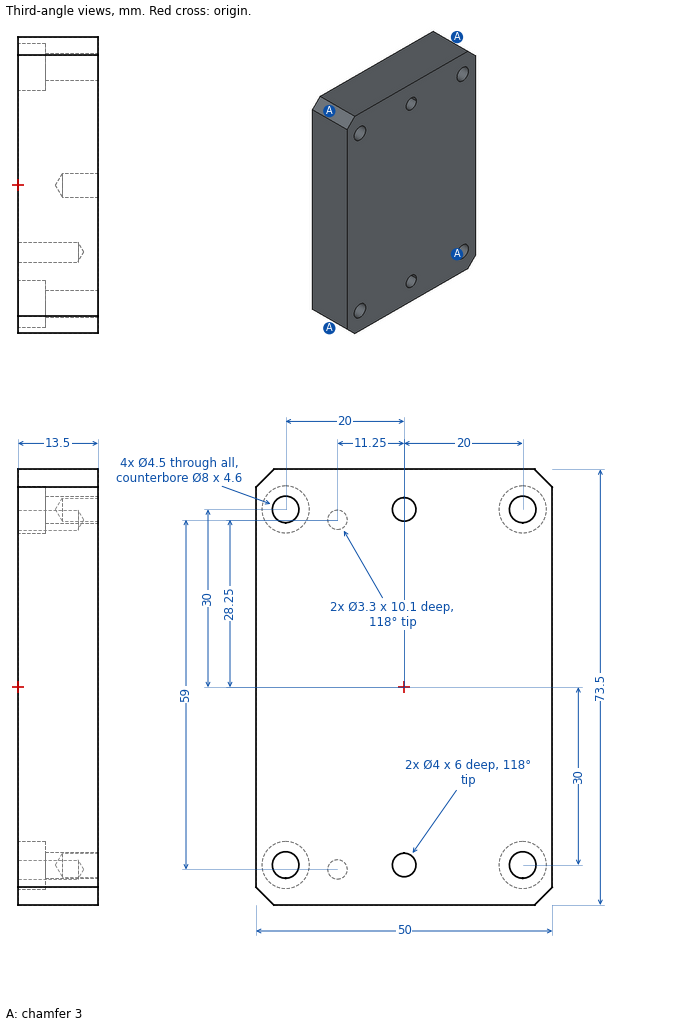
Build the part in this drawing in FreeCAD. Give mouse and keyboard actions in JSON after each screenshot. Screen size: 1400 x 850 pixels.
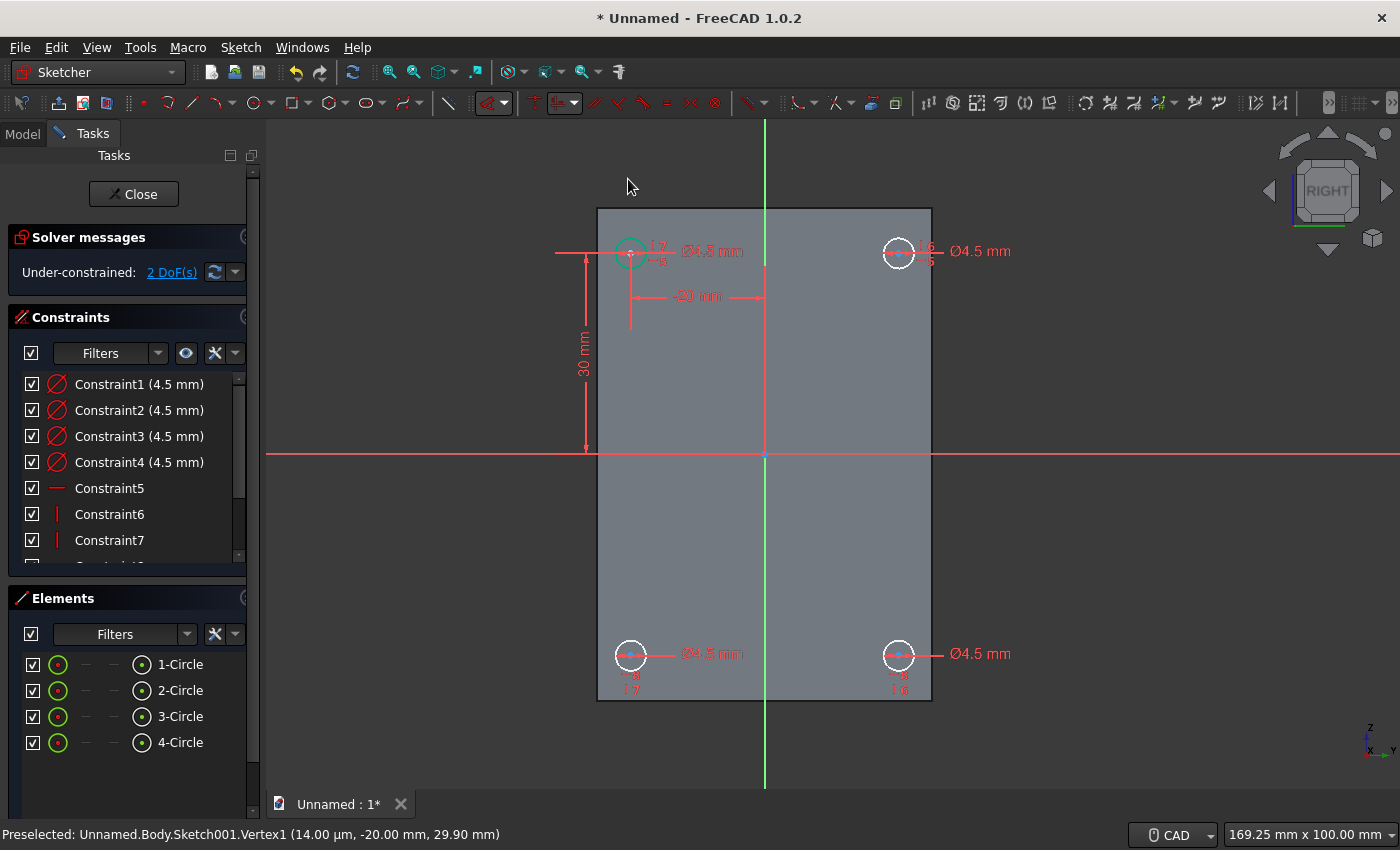
{"action": "left_click", "coordinate": [899, 253]}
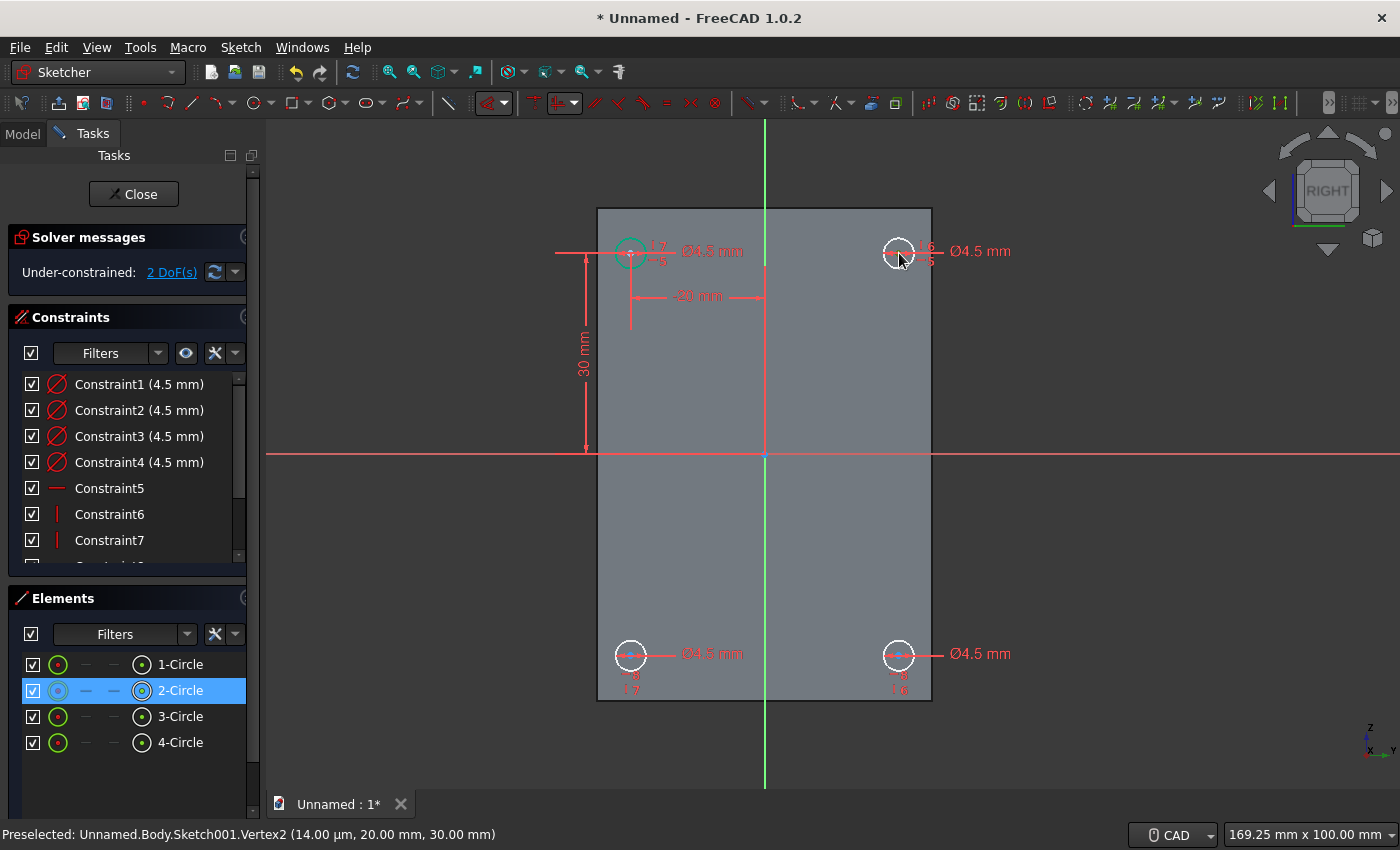
{"action": "left_click", "coordinate": [506, 104]}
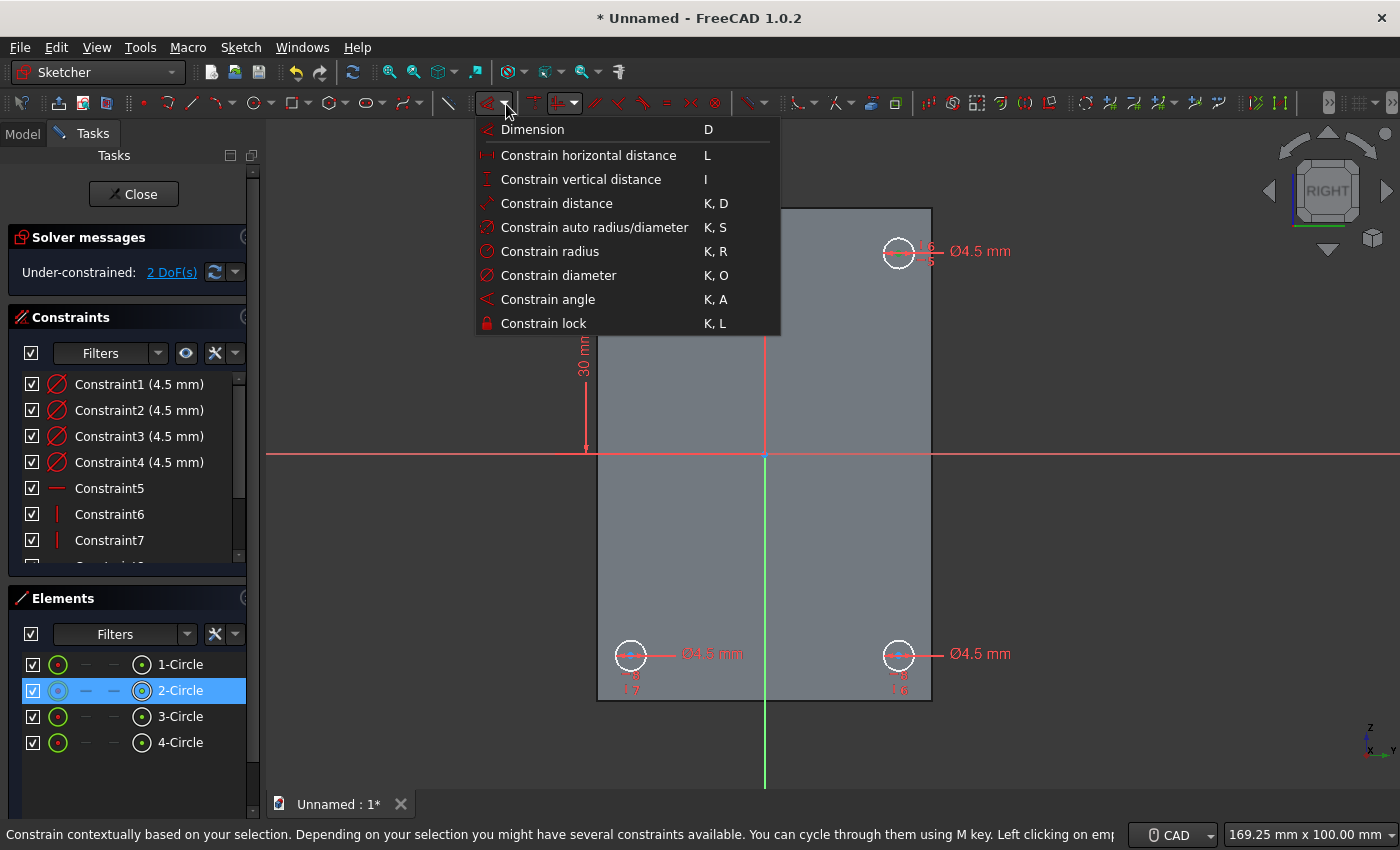
{"action": "left_click", "coordinate": [628, 155]}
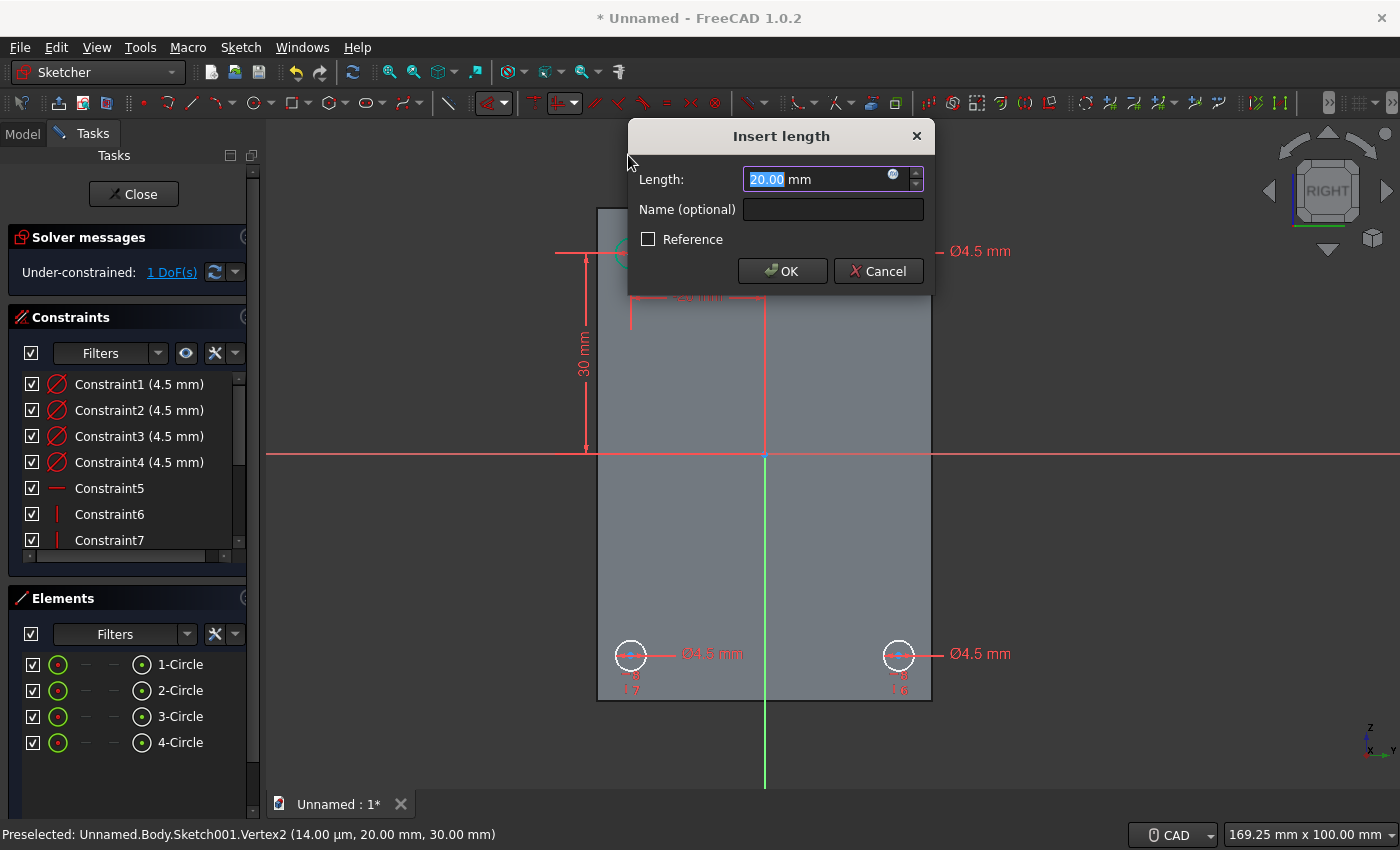
{"action": "type", "text": "20"}
{"action": "key", "text": "Return"}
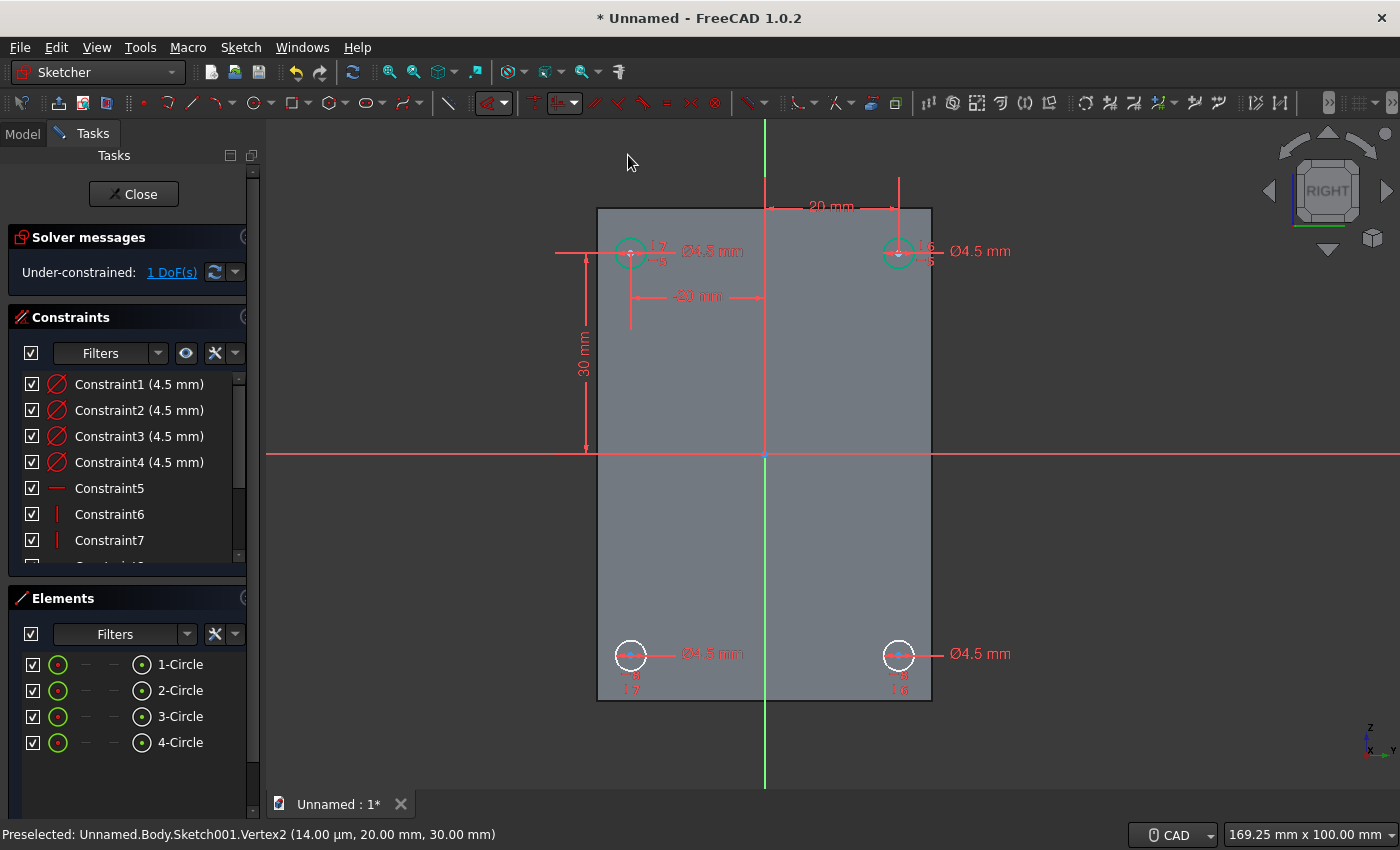
{"action": "left_click", "coordinate": [899, 656]}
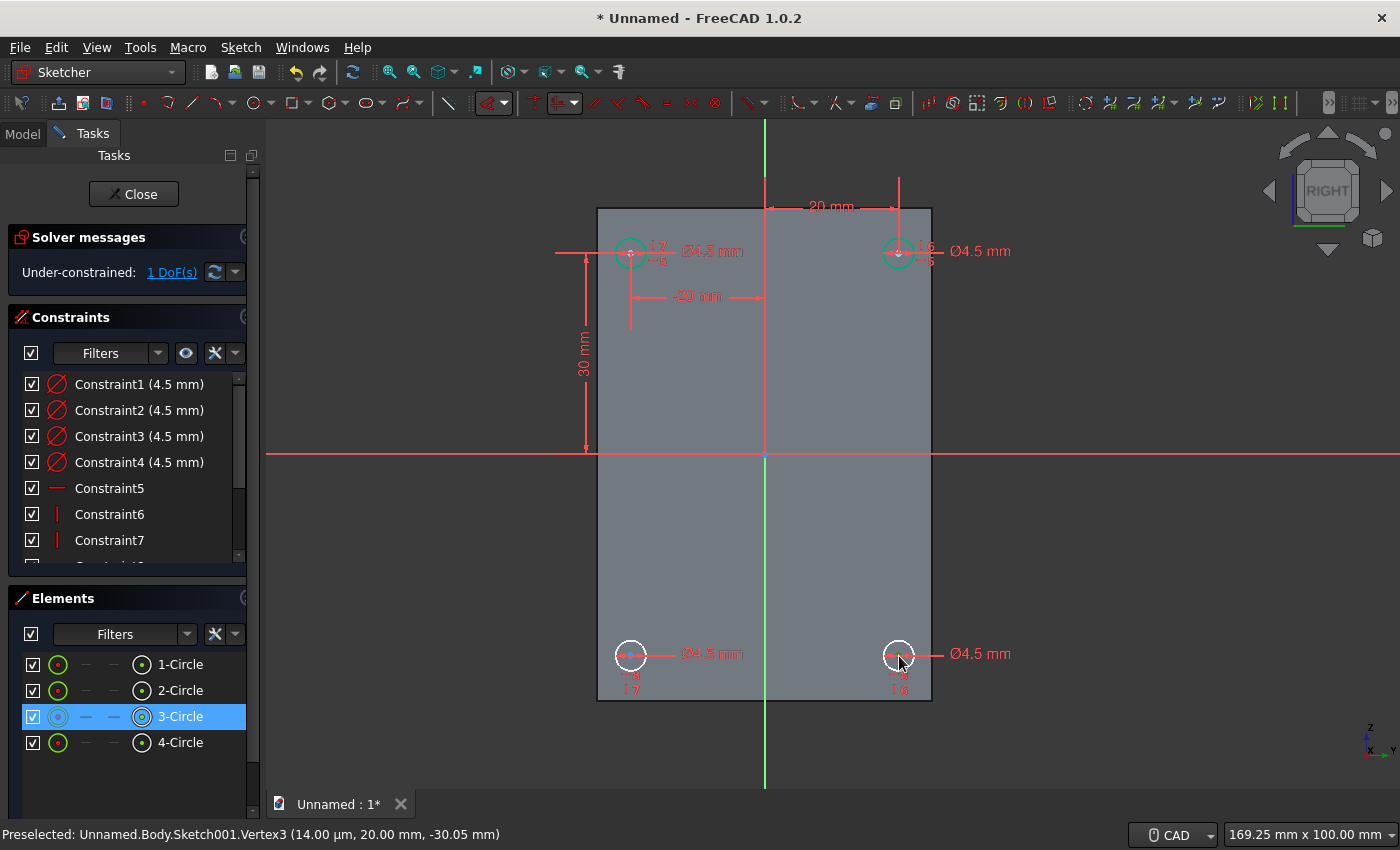
{"action": "left_click", "coordinate": [506, 104]}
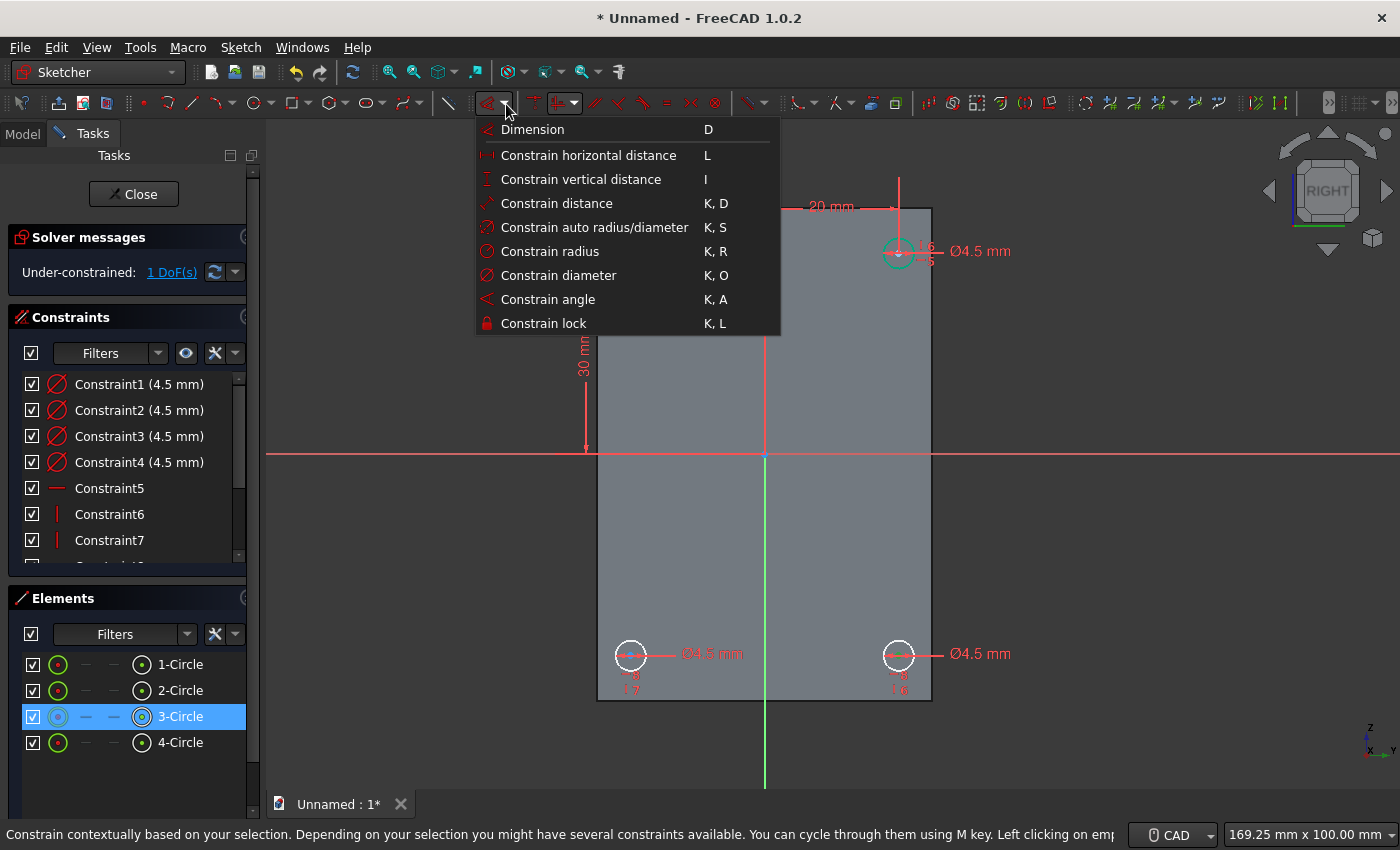
{"action": "left_click", "coordinate": [628, 179]}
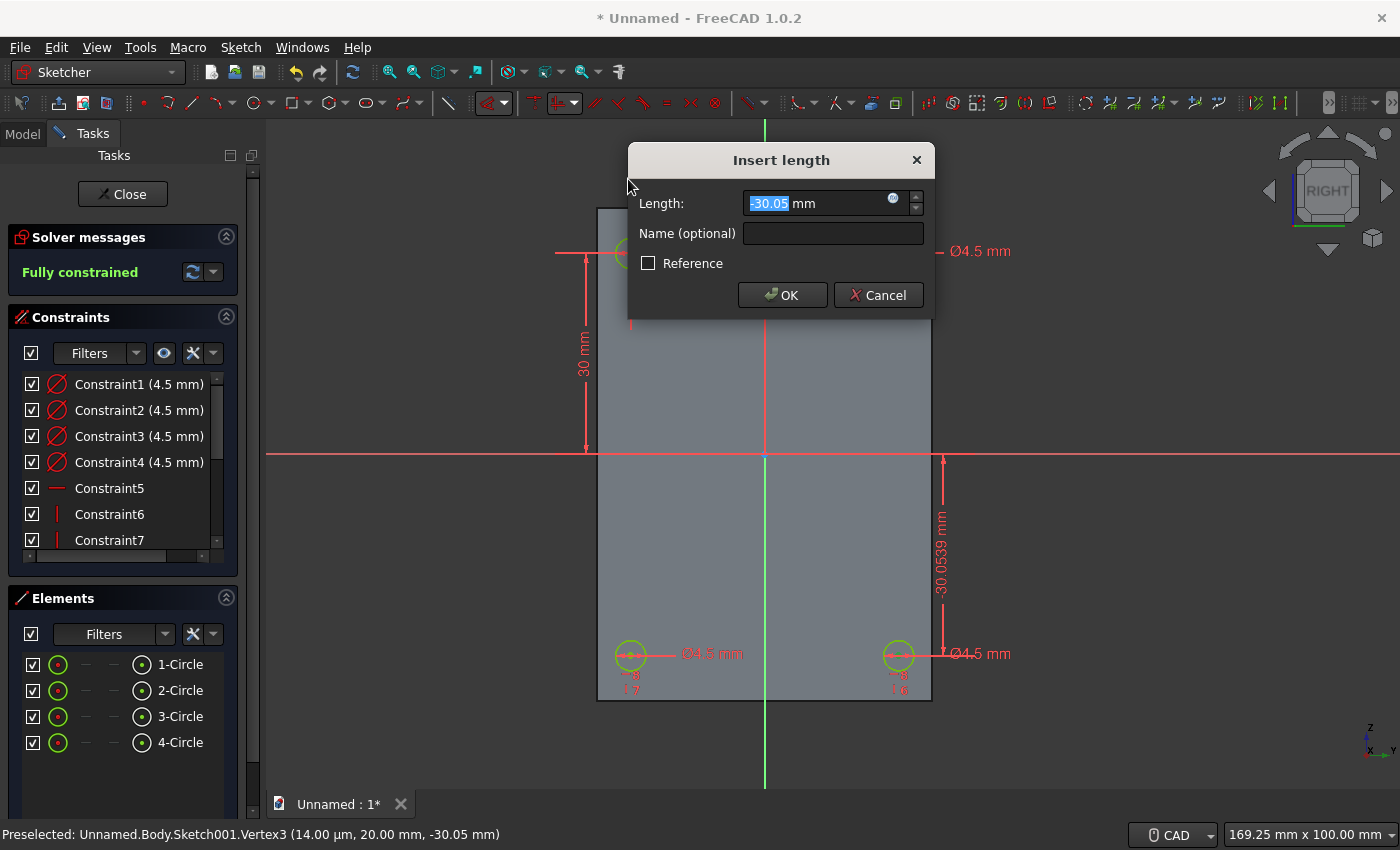
{"action": "type", "text": "-30"}
{"action": "key", "text": "Return"}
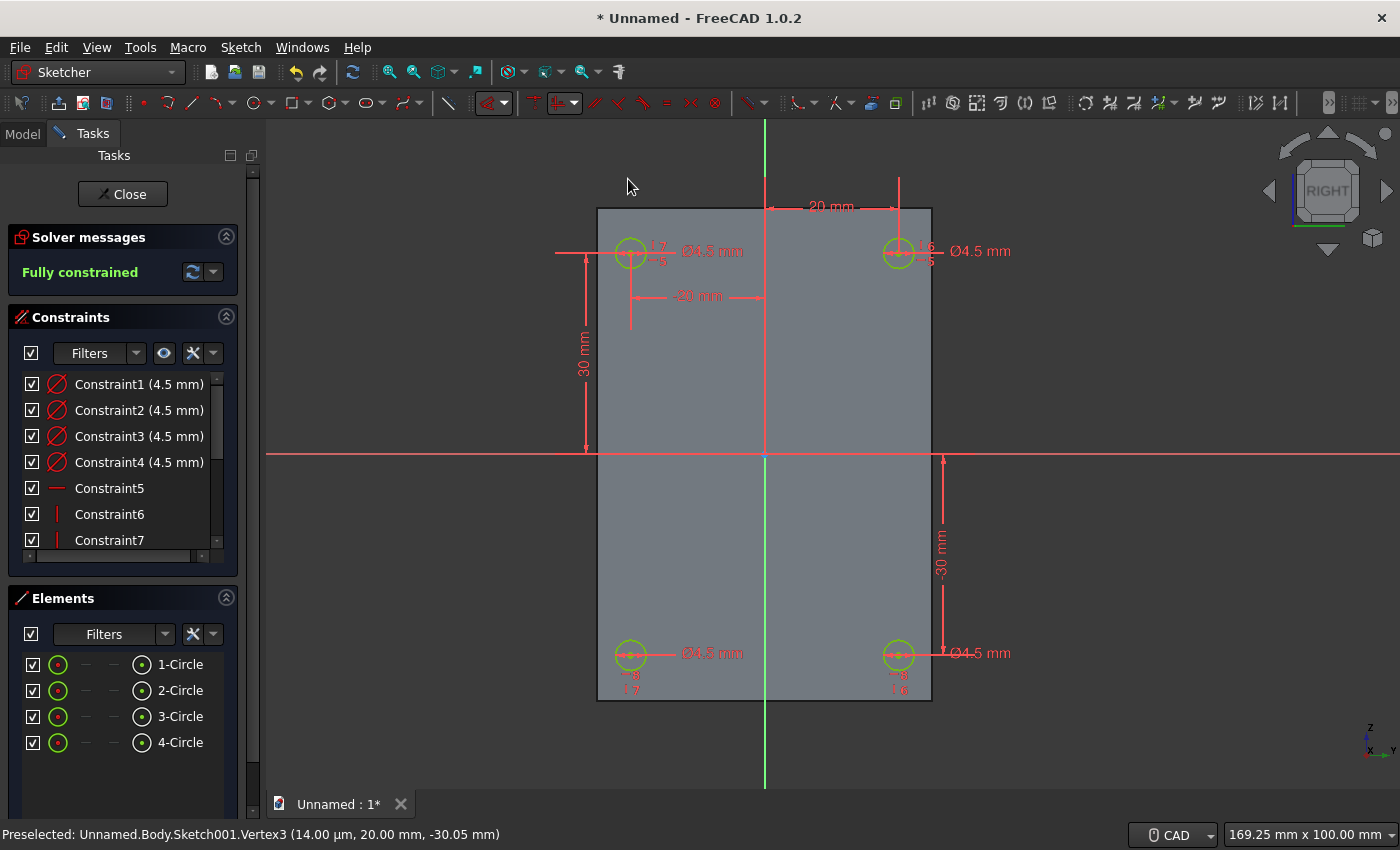
{"action": "left_click", "coordinate": [123, 194]}